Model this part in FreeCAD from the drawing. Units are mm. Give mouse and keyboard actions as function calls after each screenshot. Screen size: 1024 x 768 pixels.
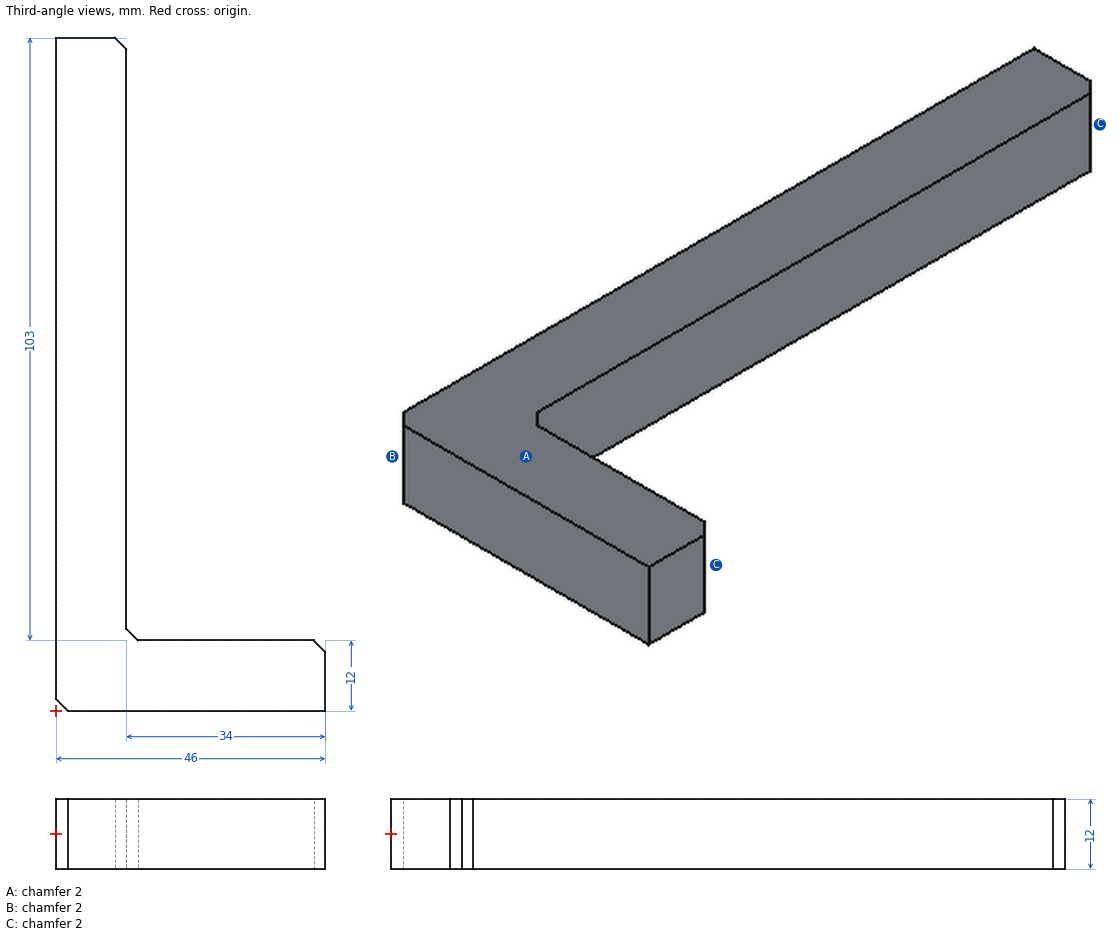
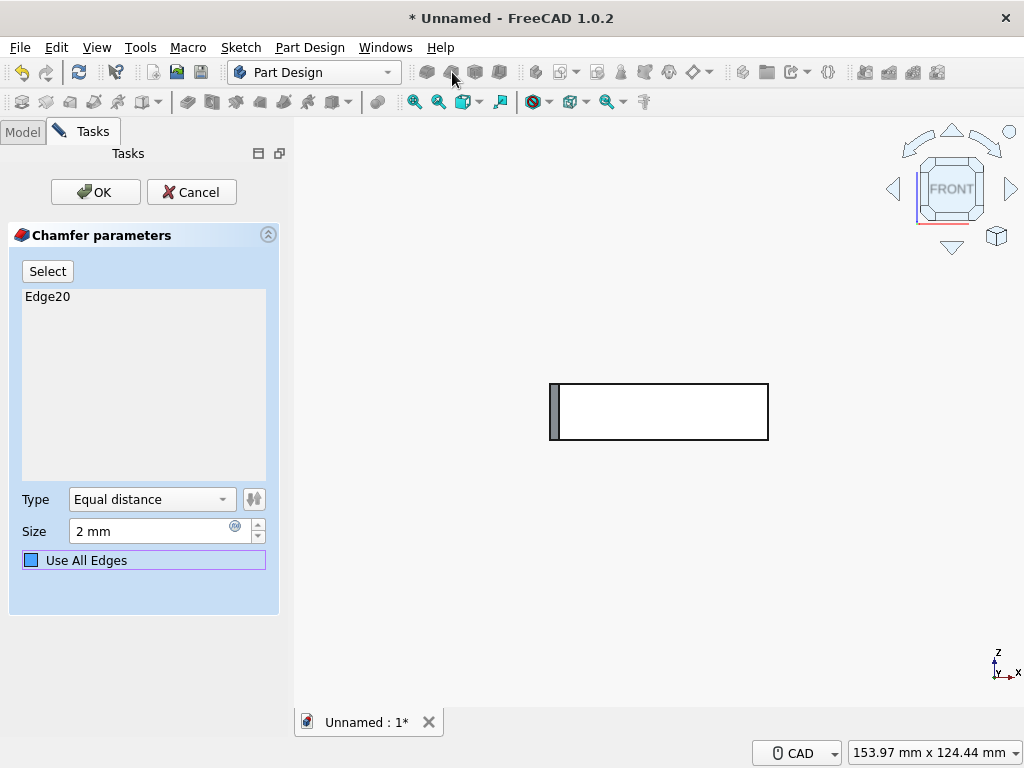
click(96, 192)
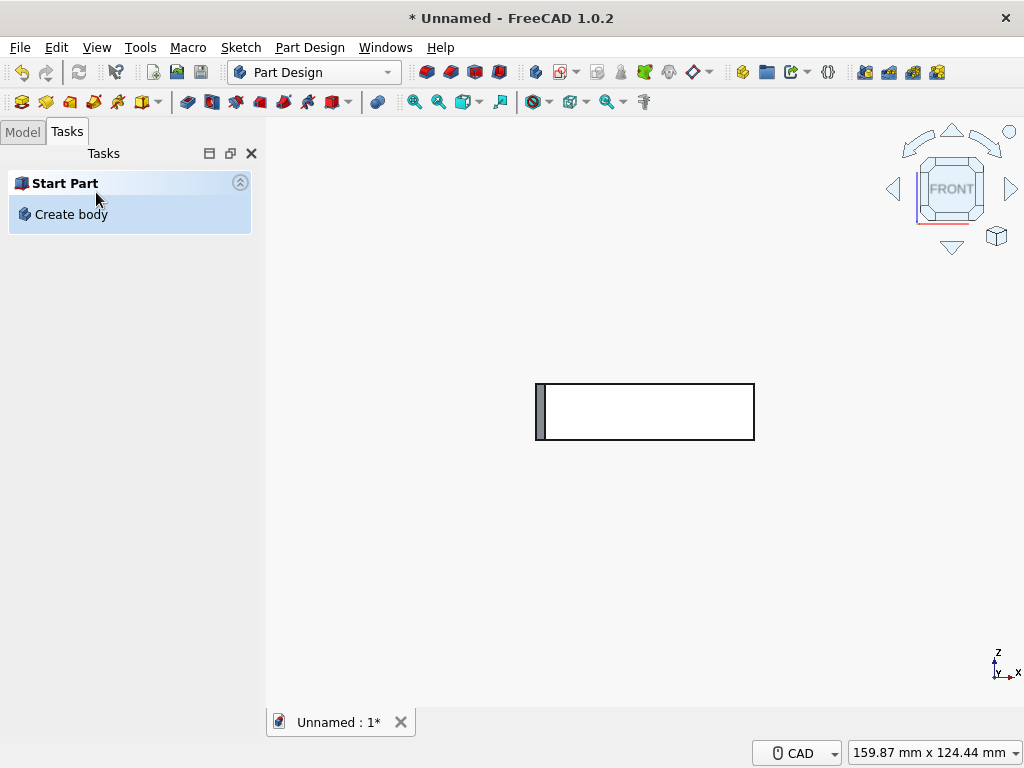
click(416, 102)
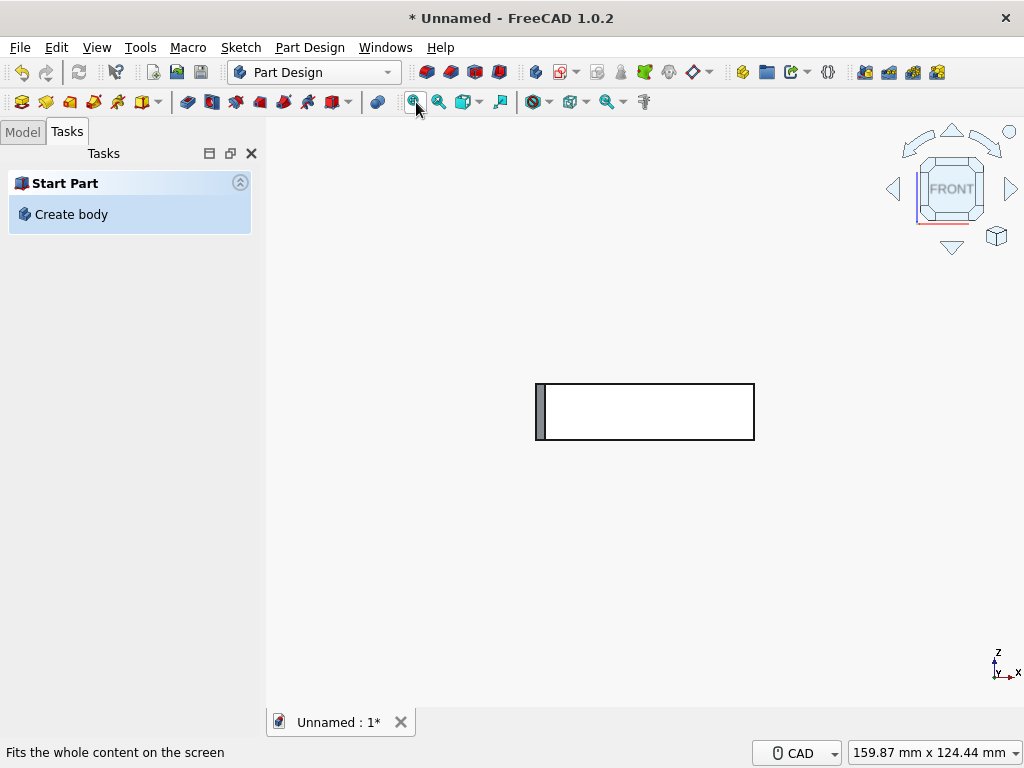
key(0)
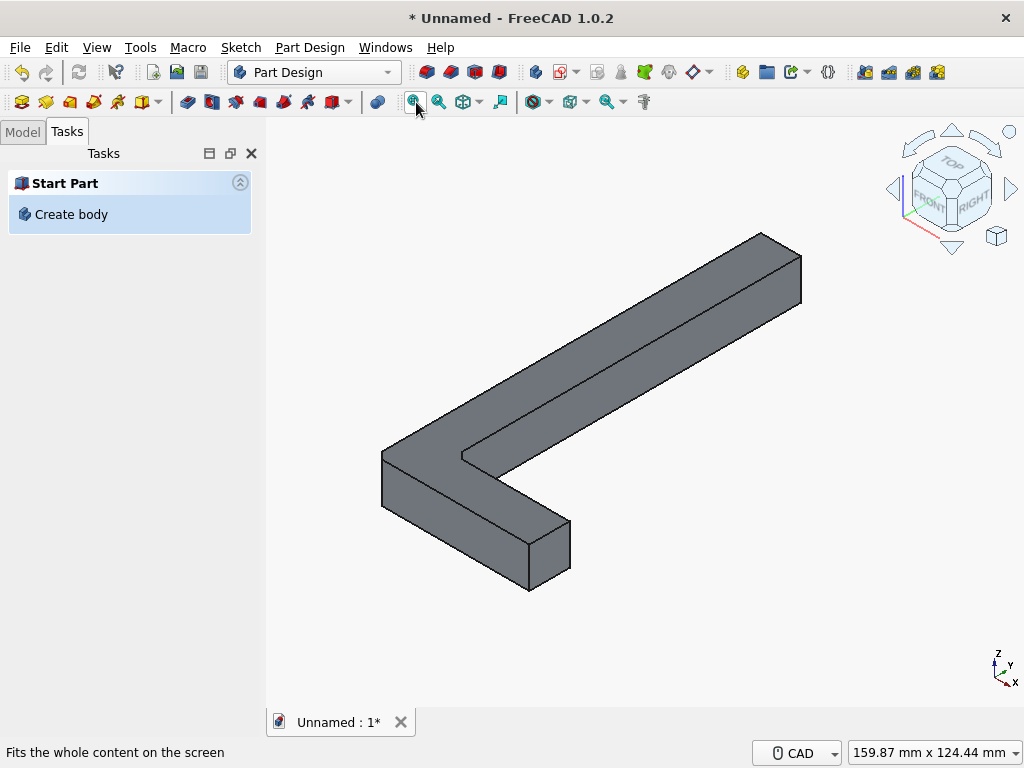
key(2)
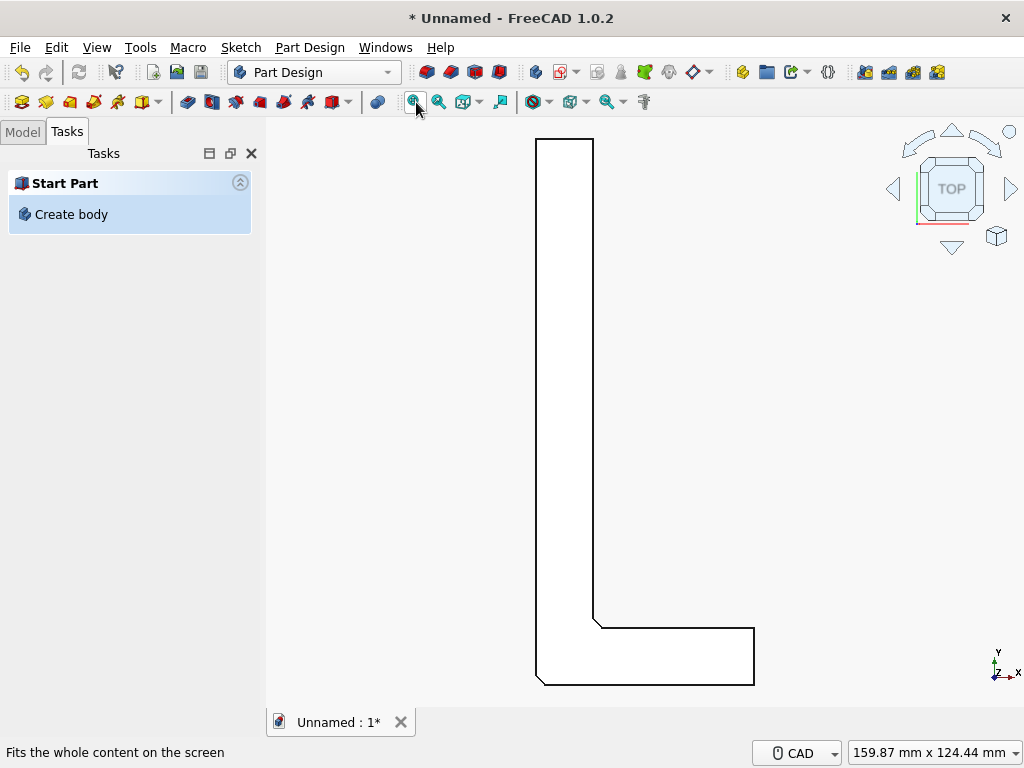
key(1)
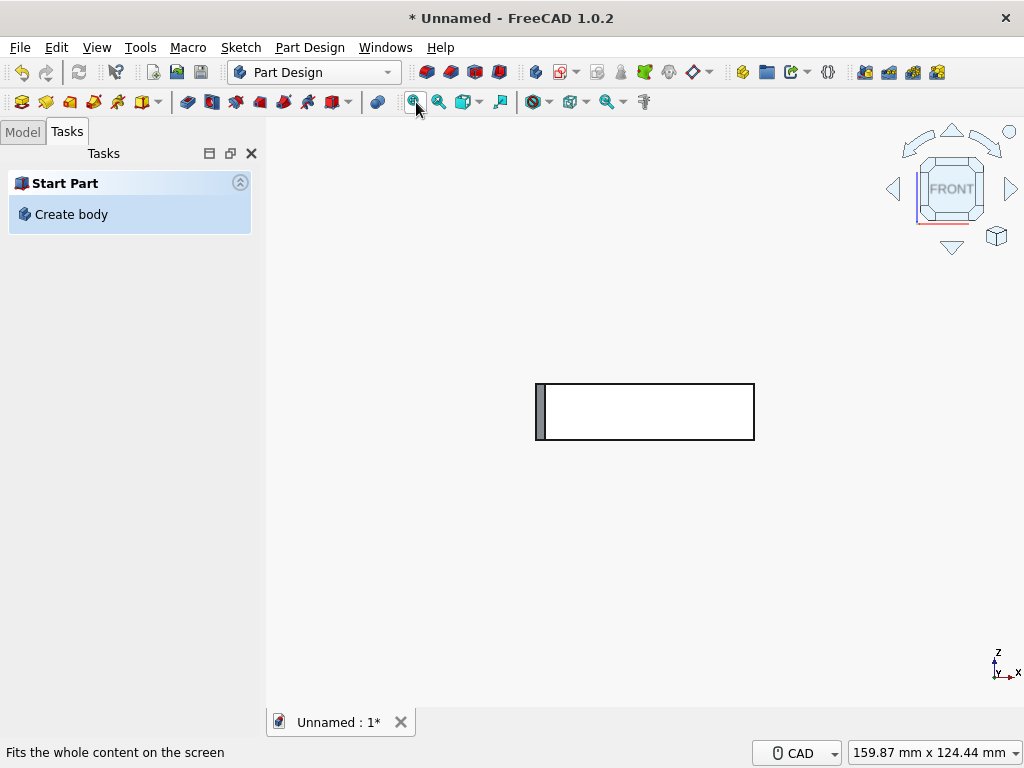
key(v)
key(f)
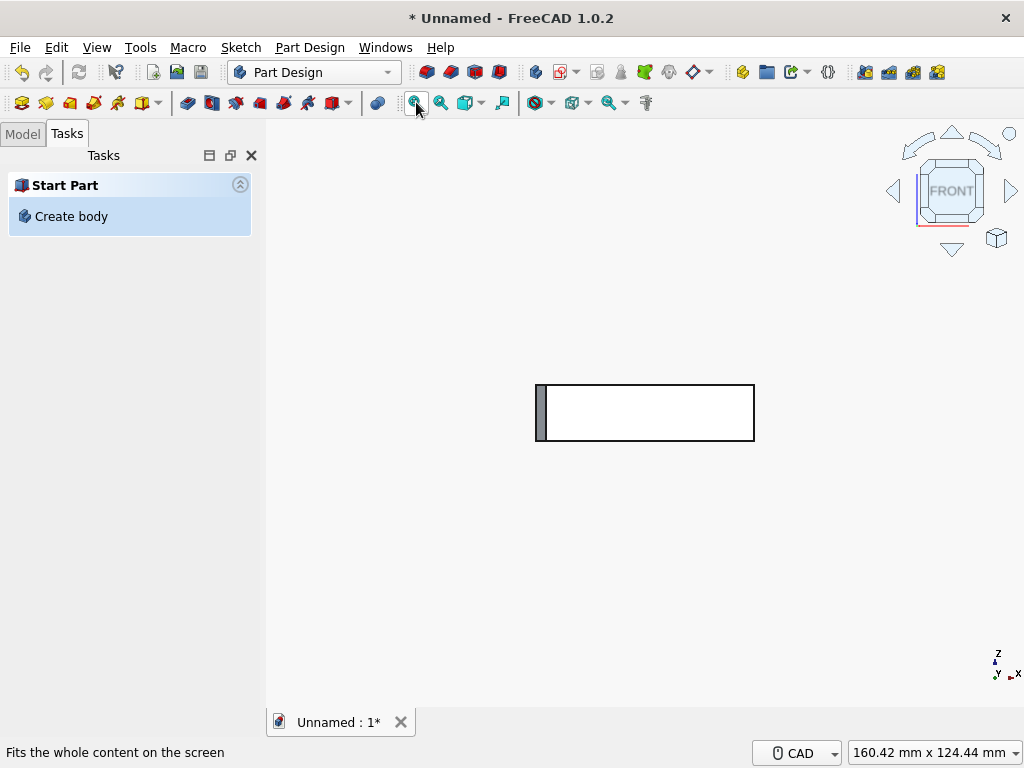
key(3)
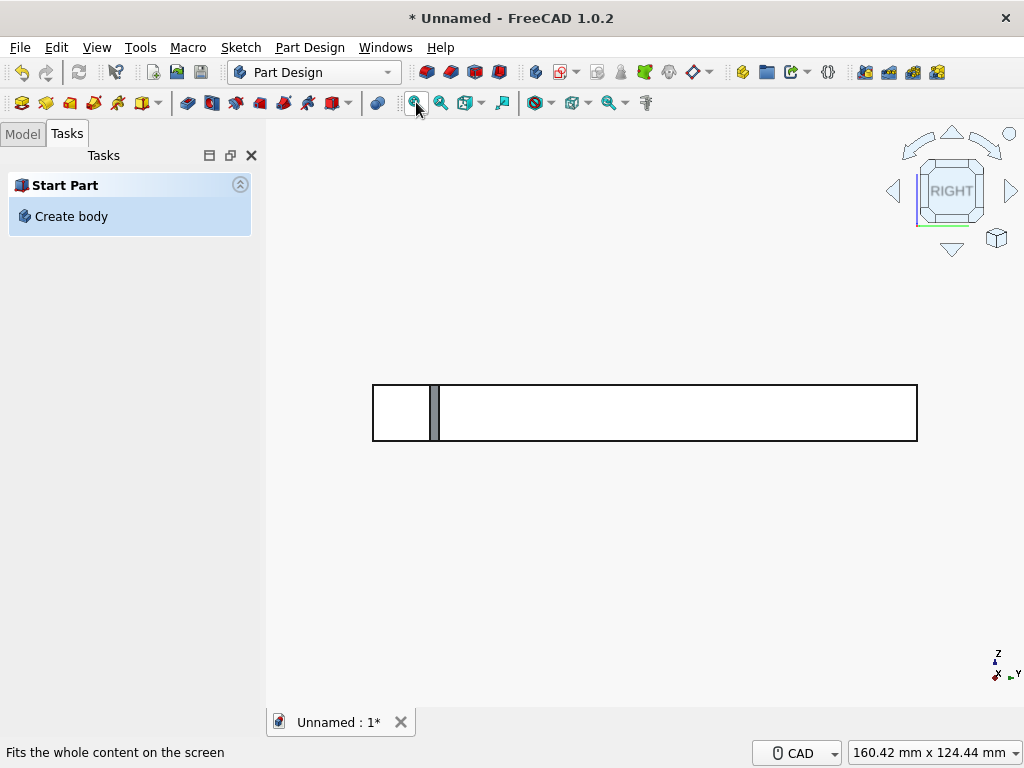
click(917, 412)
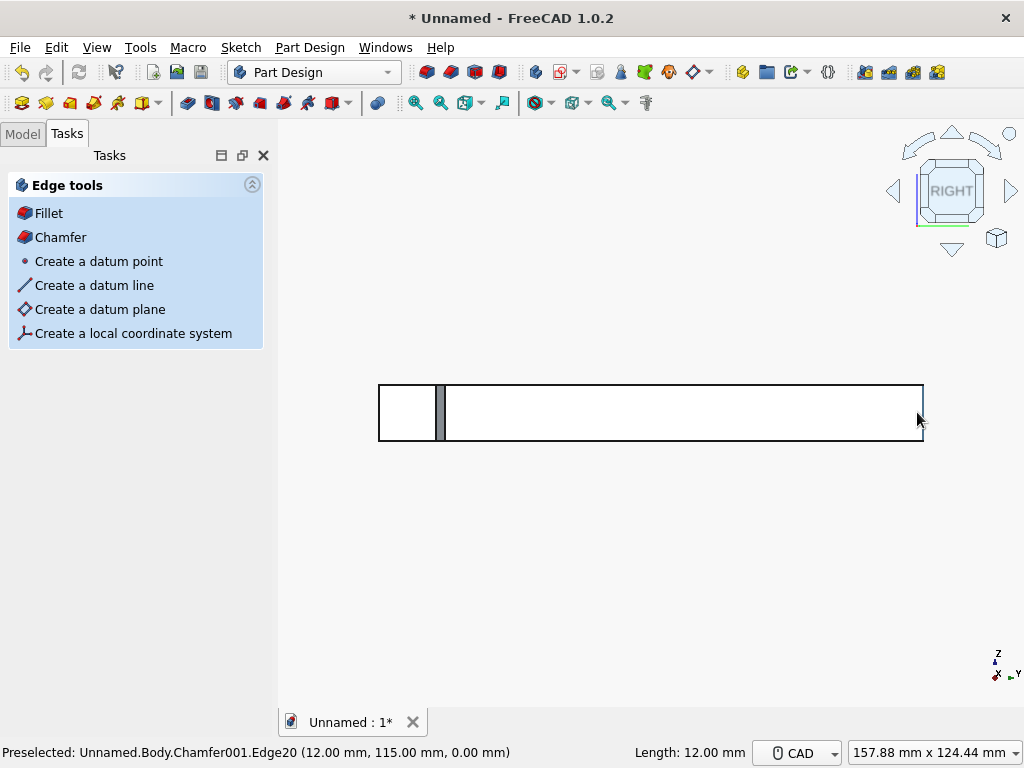
click(436, 412, ctrl)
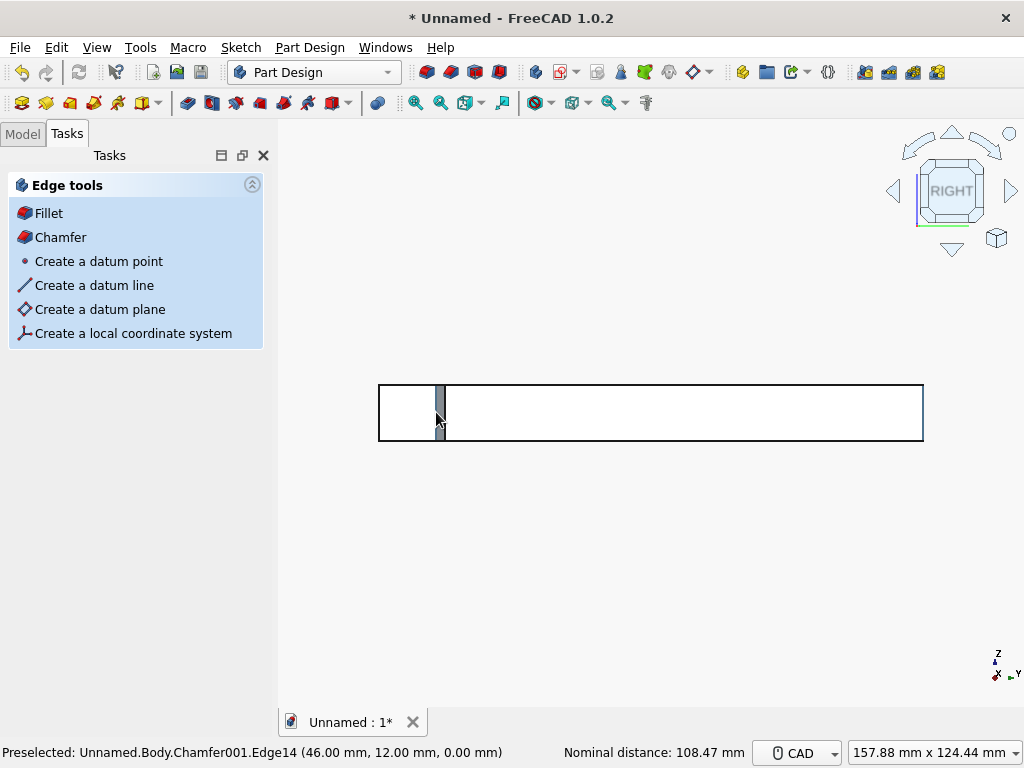
click(452, 72)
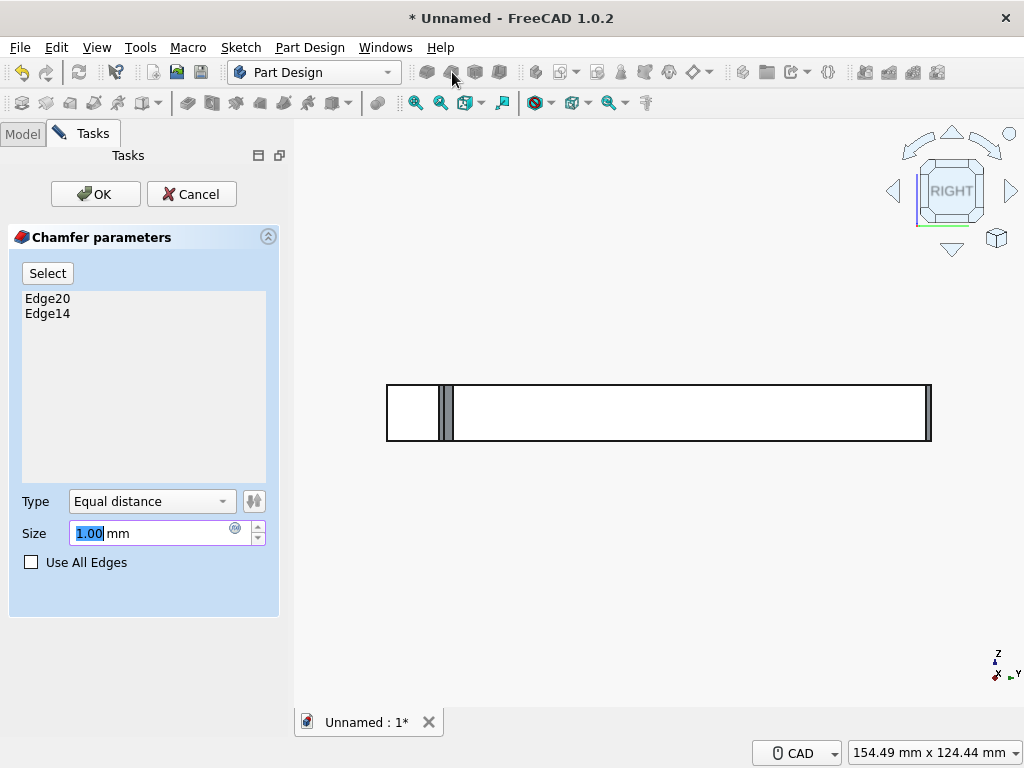
text(2)
key(Tab)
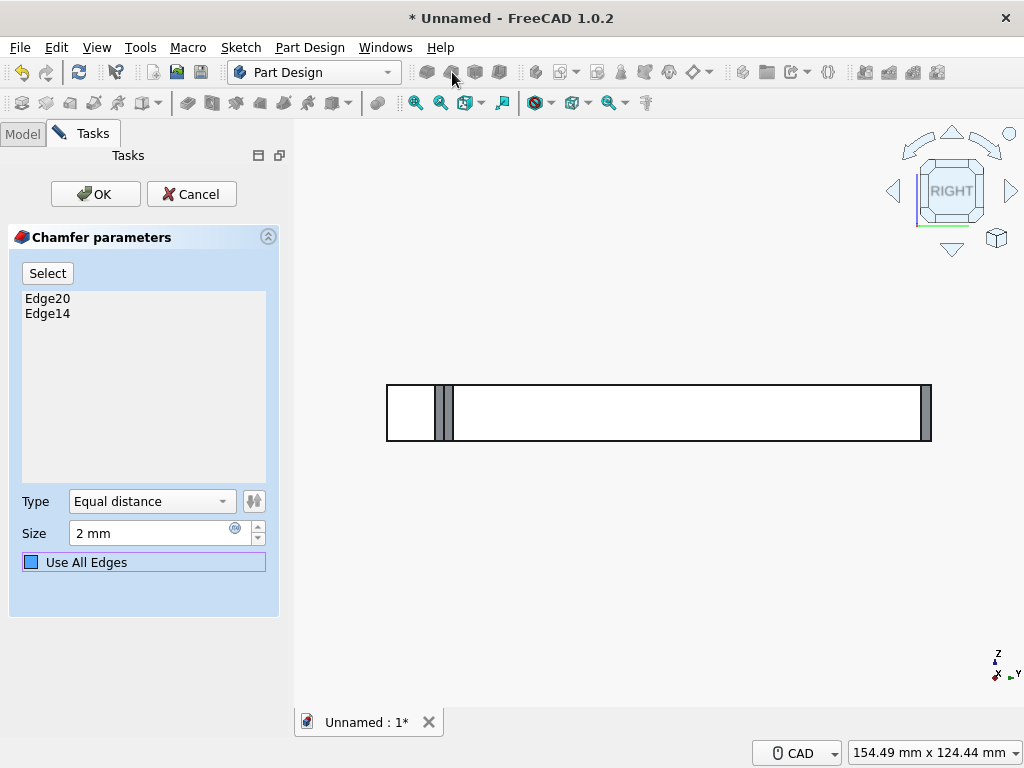
click(96, 194)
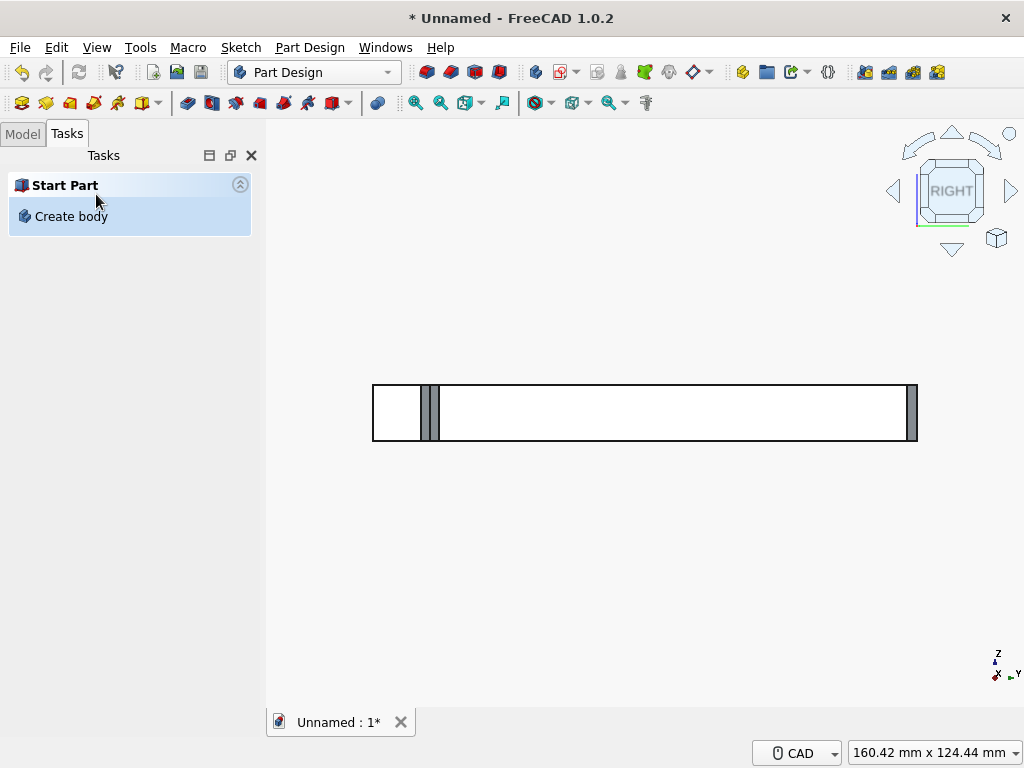
key(0)